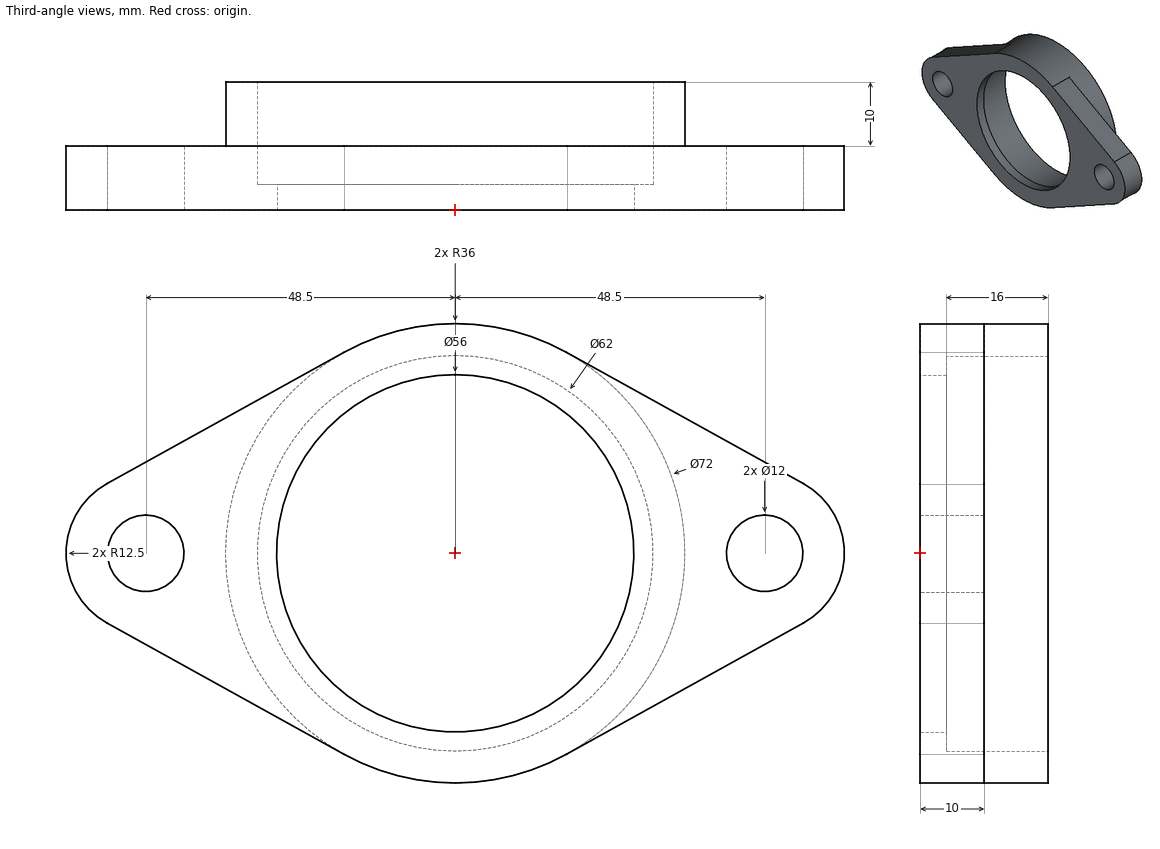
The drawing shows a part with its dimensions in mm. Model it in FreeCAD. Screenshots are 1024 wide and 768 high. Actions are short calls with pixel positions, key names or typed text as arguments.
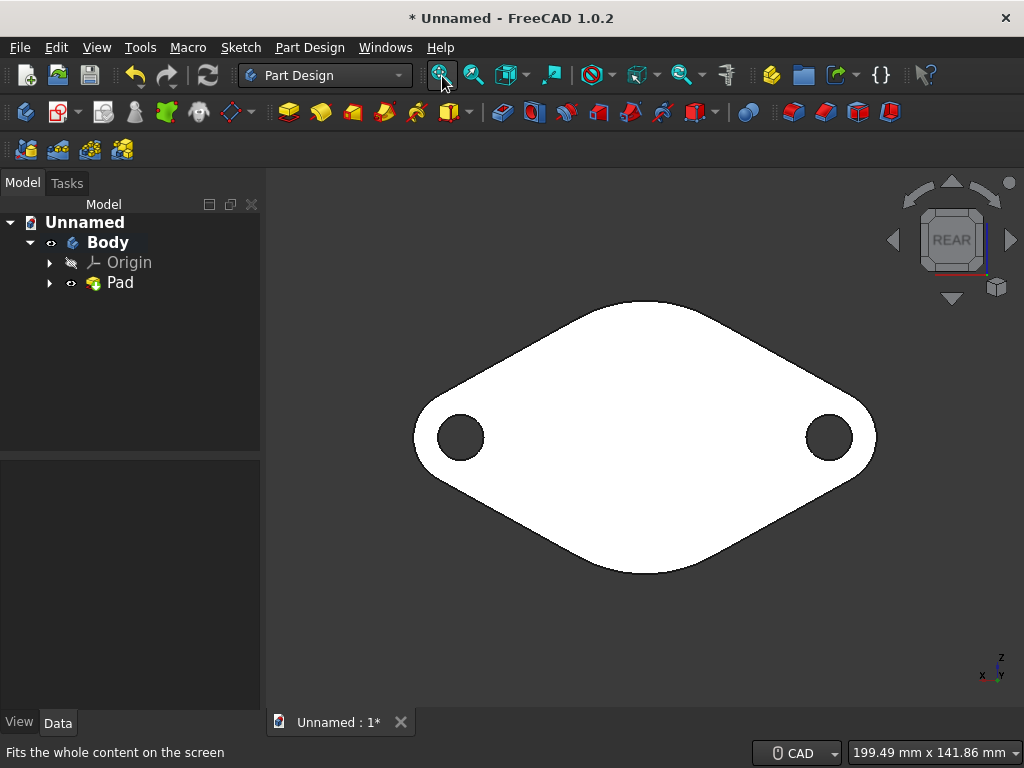
click(645, 437)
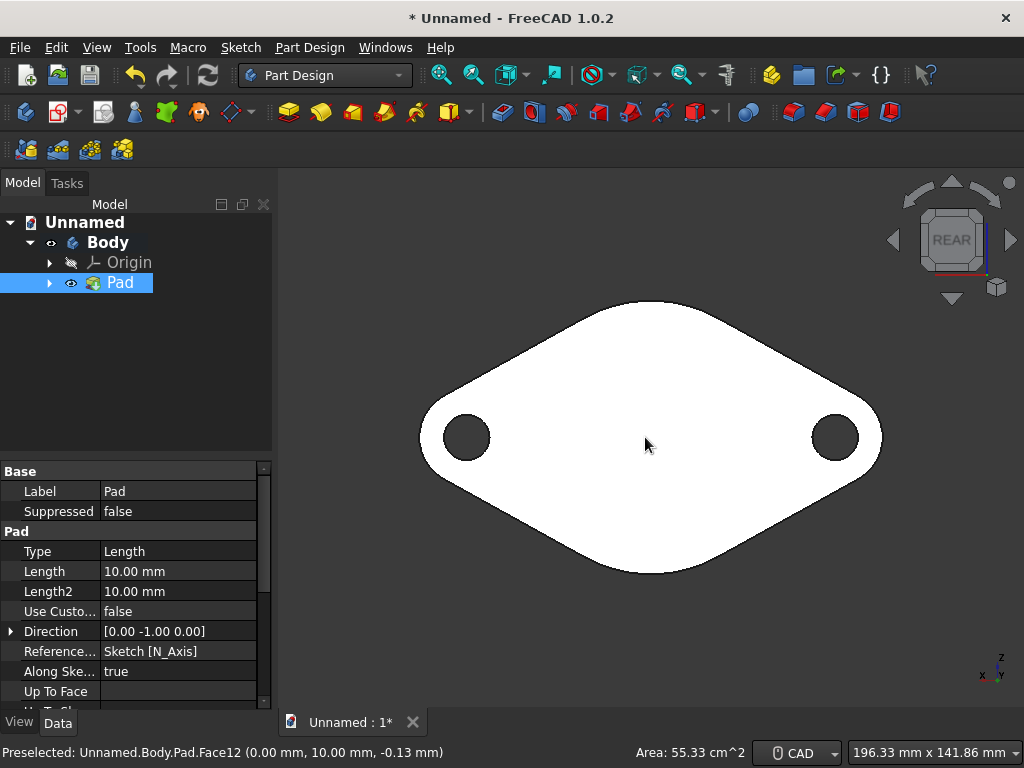
click(58, 112)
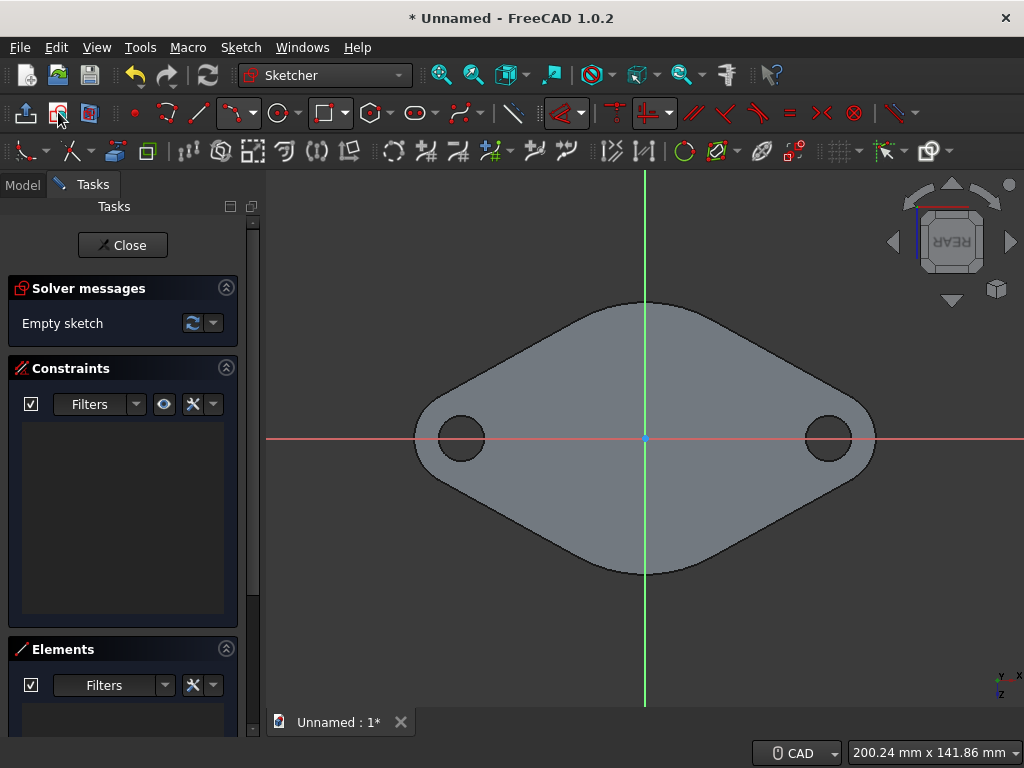
click(278, 114)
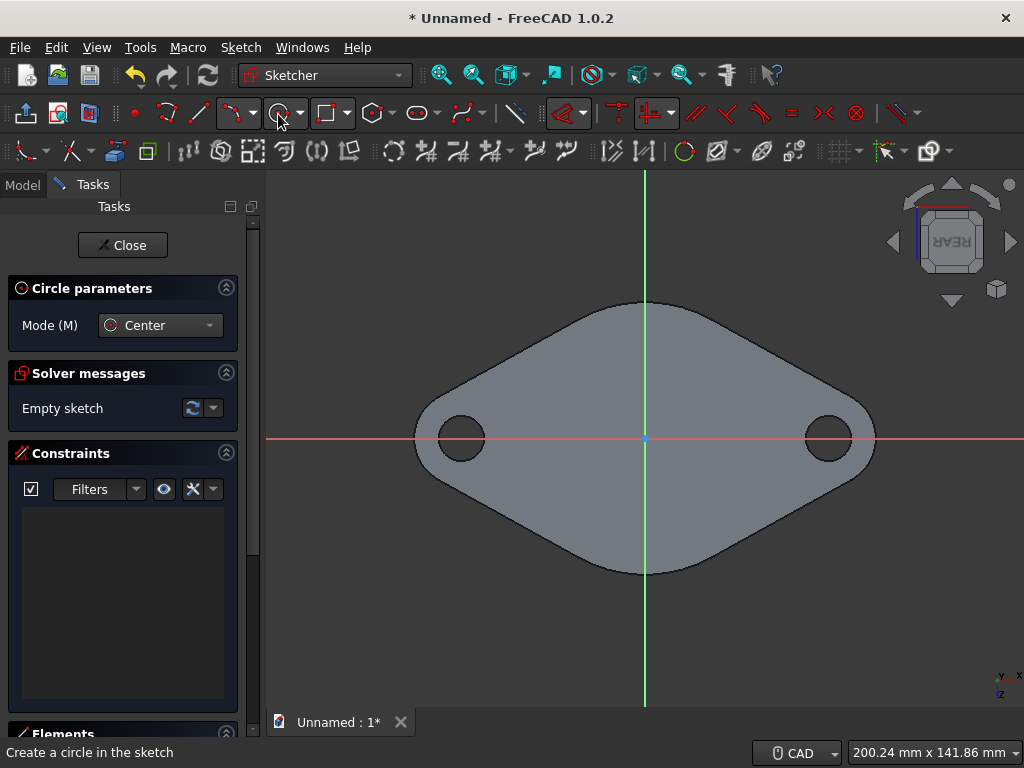
click(645, 438)
click(741, 342)
key(Escape)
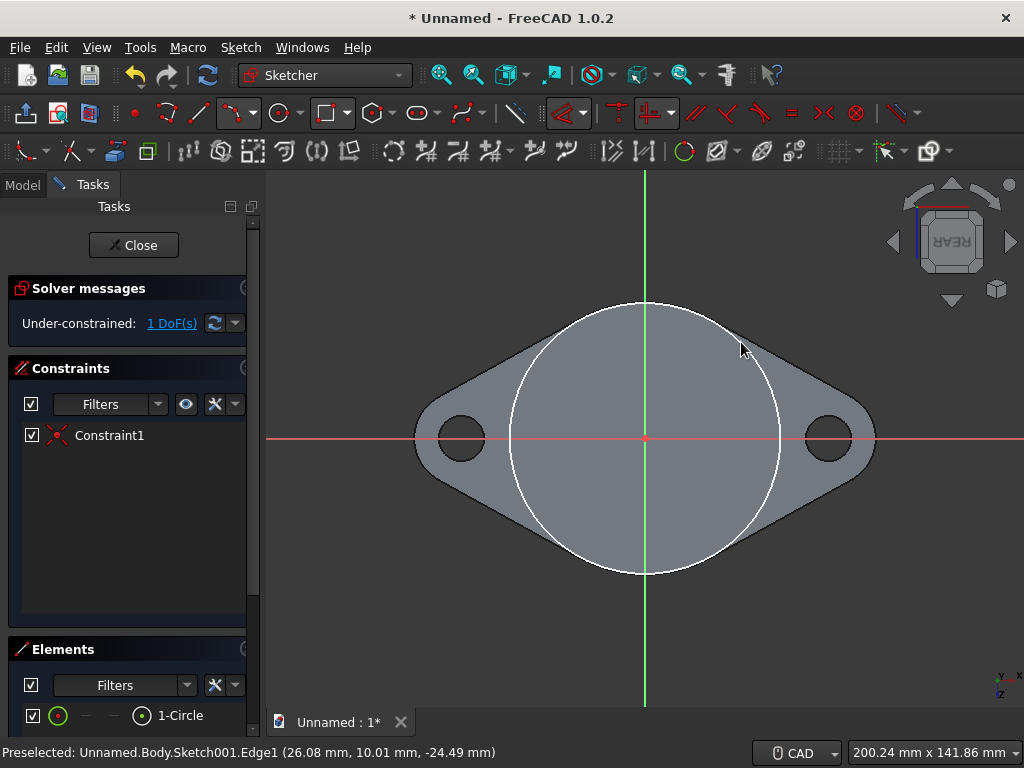
click(740, 342)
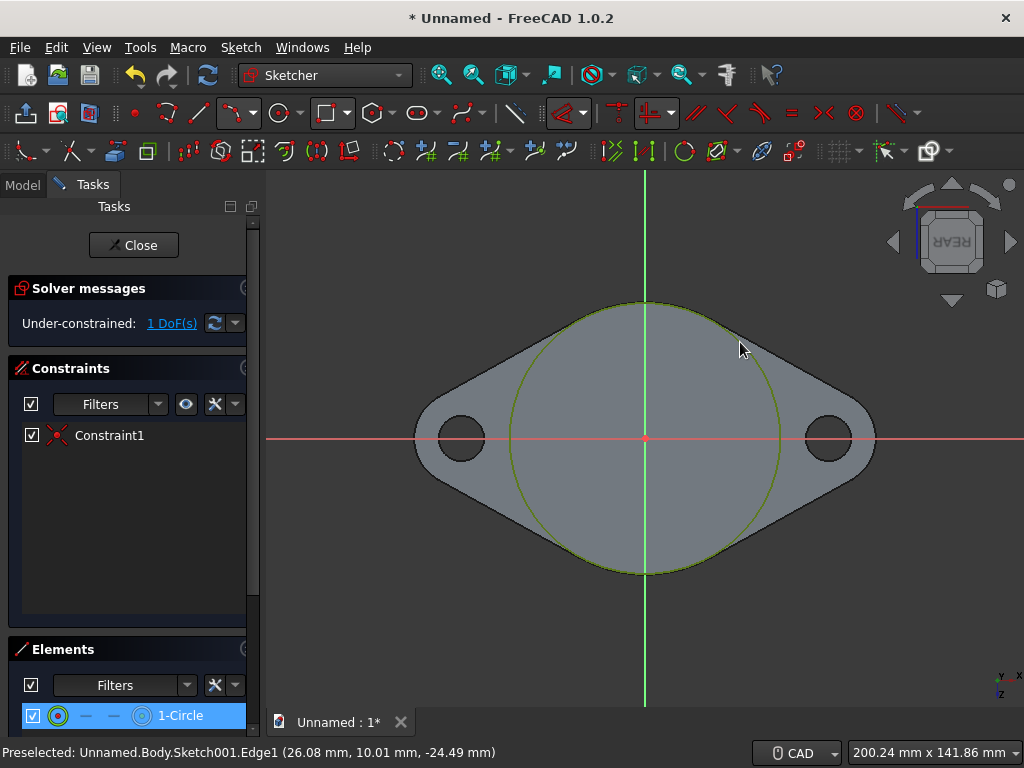
key(k)
key(o)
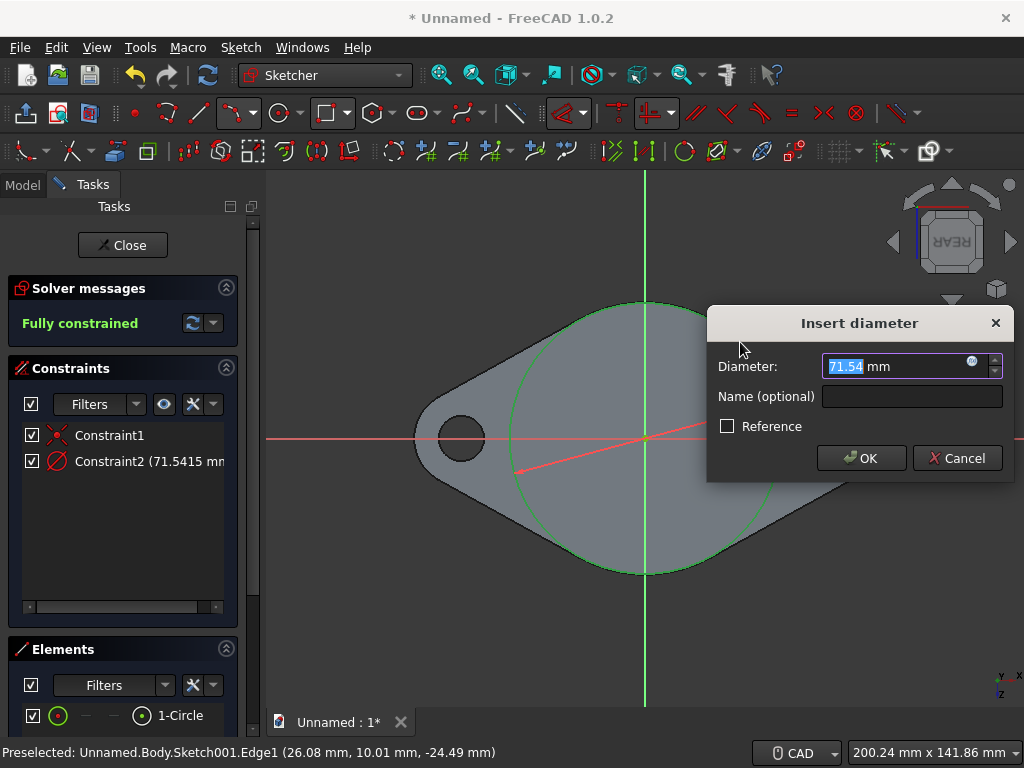
text(72)
key(Return)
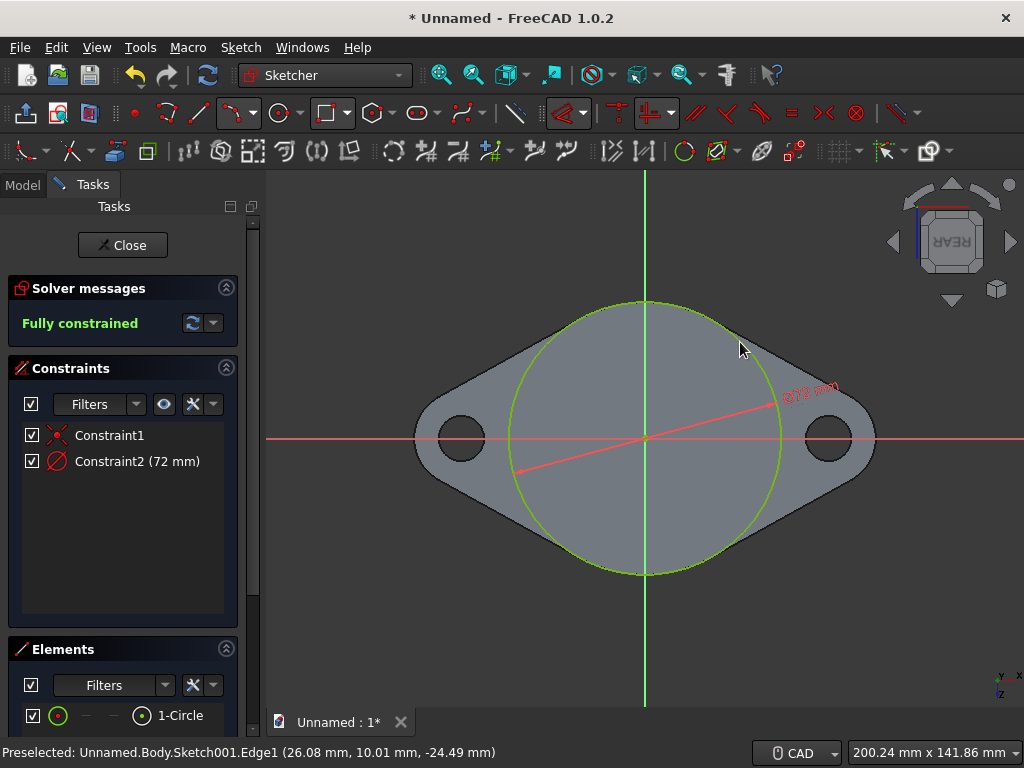
click(123, 245)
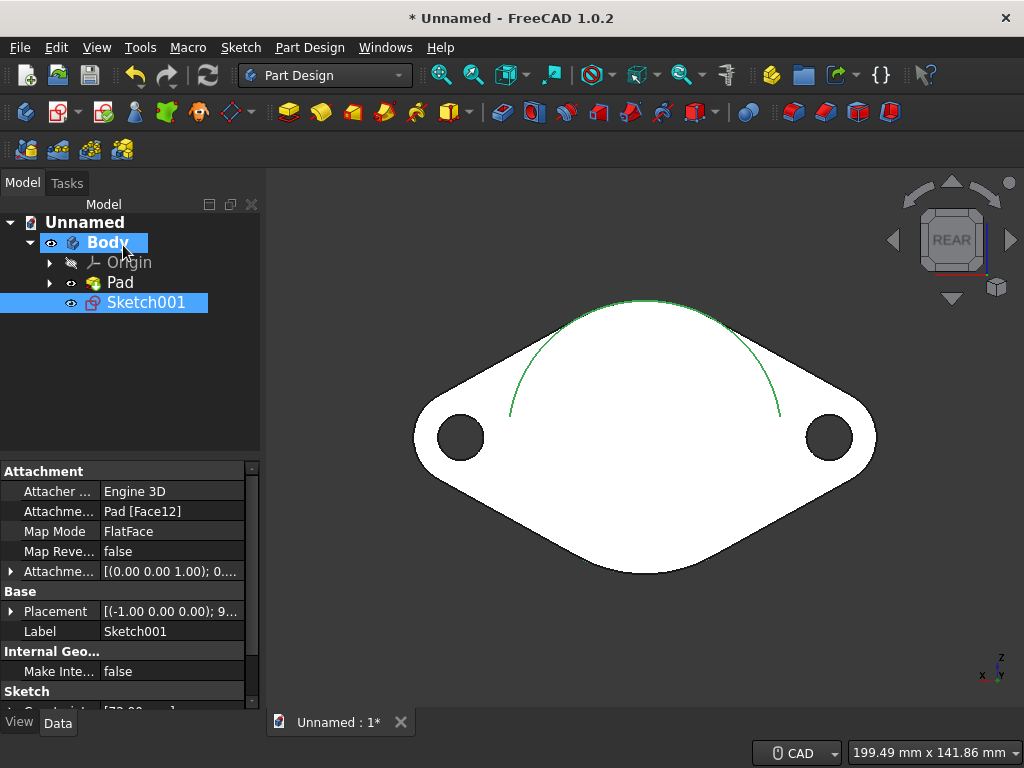
click(290, 112)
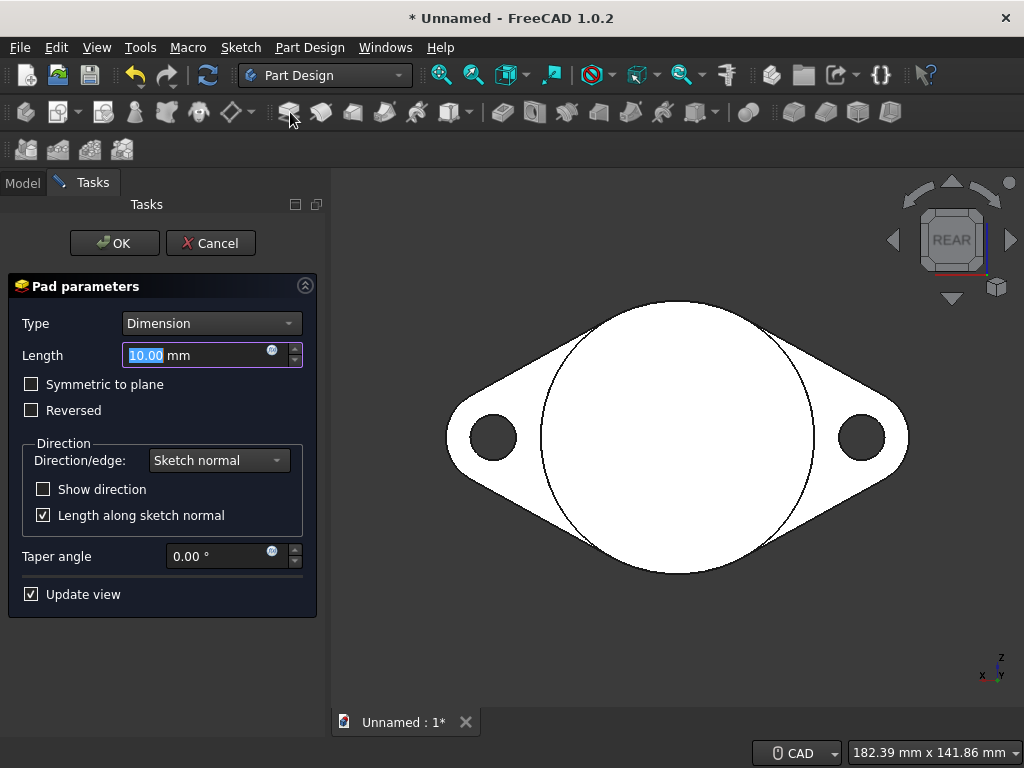
text(10)
key(Tab)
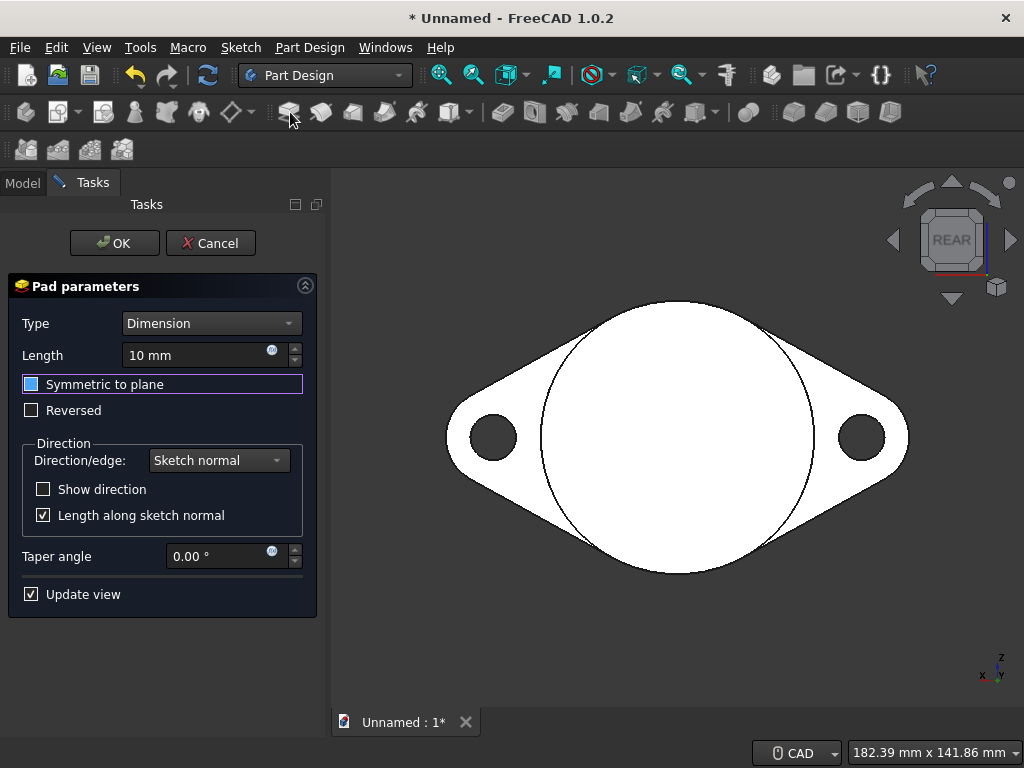
click(115, 243)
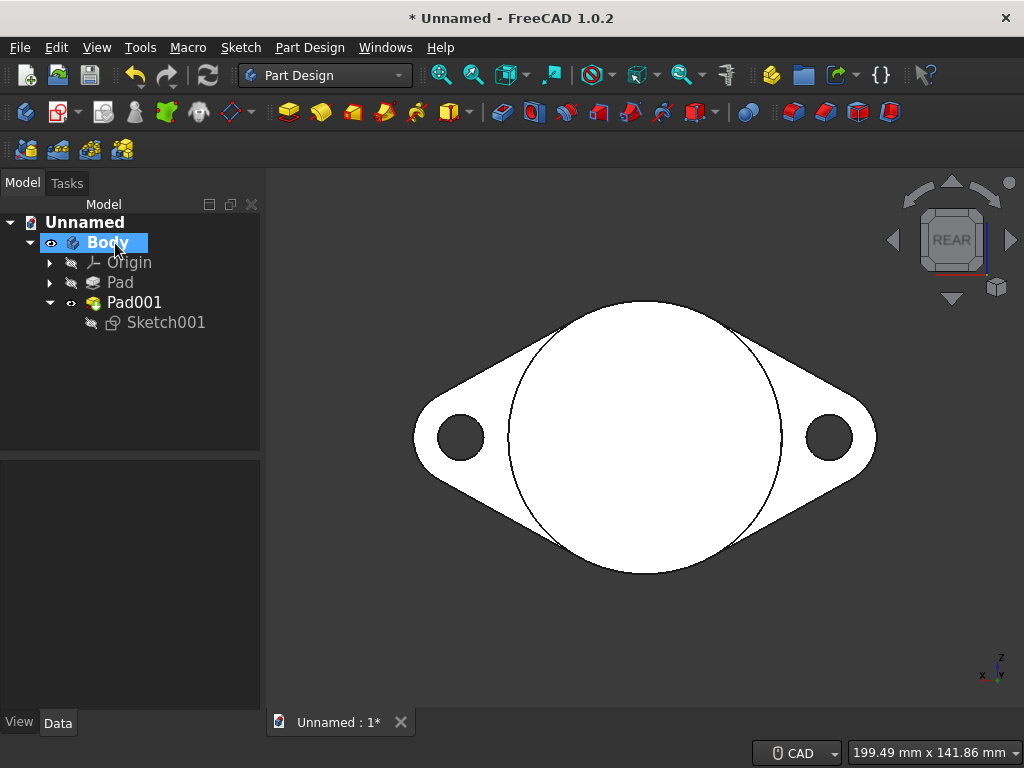
click(645, 437)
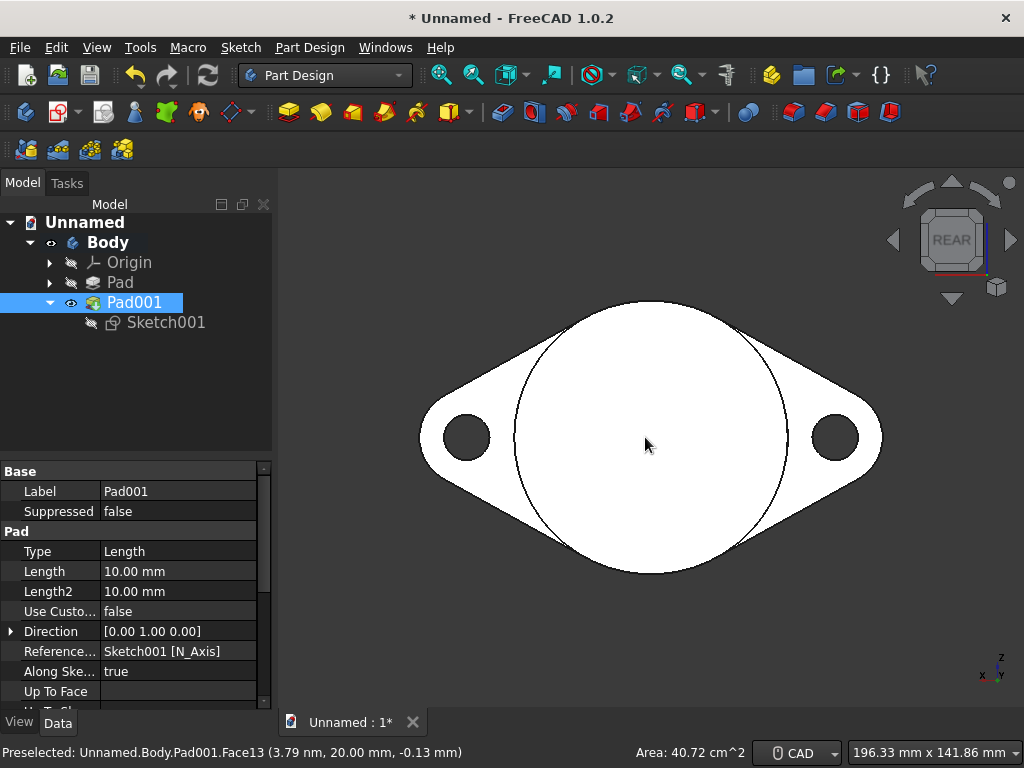
click(58, 112)